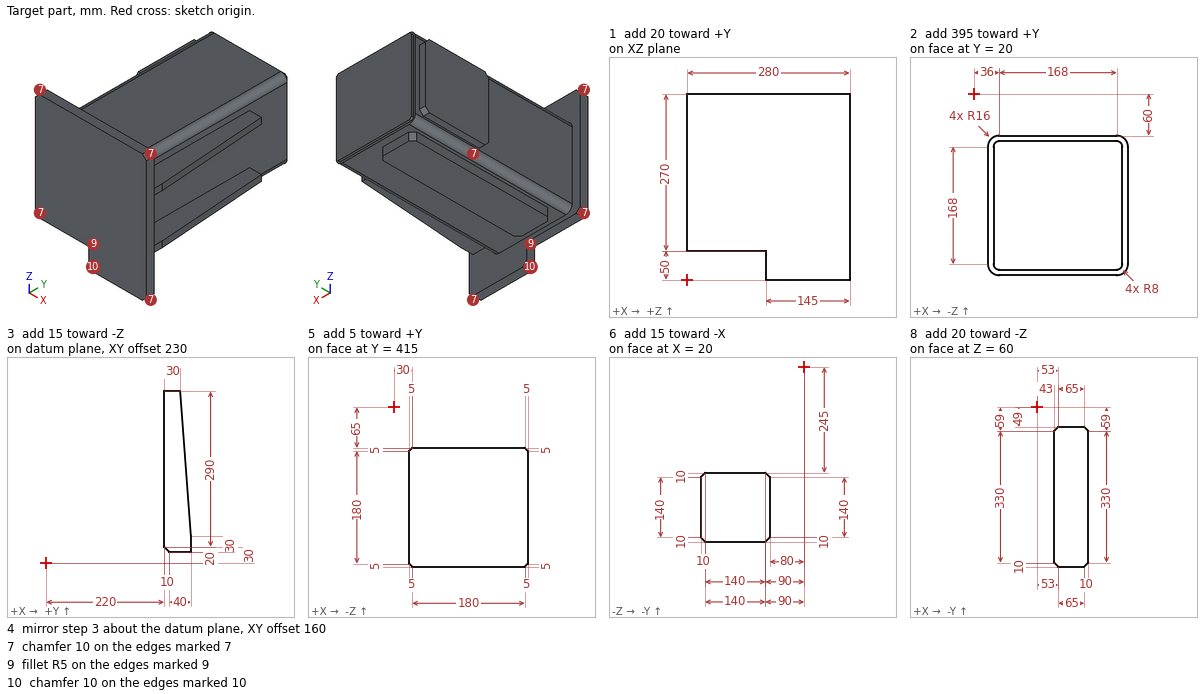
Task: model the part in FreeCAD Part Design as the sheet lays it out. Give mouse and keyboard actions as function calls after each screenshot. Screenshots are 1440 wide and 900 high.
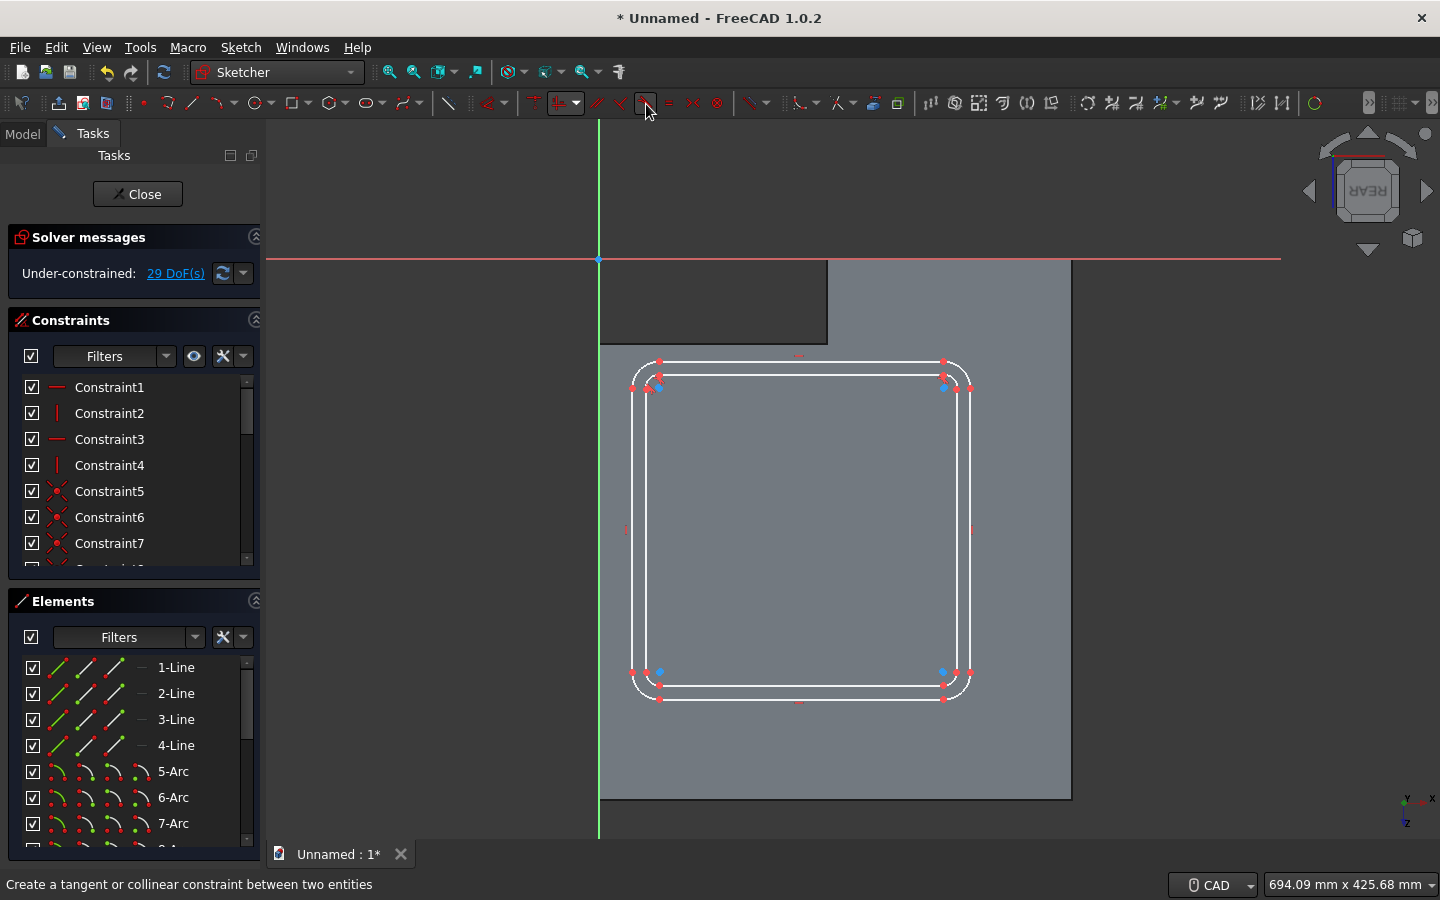
click(632, 474)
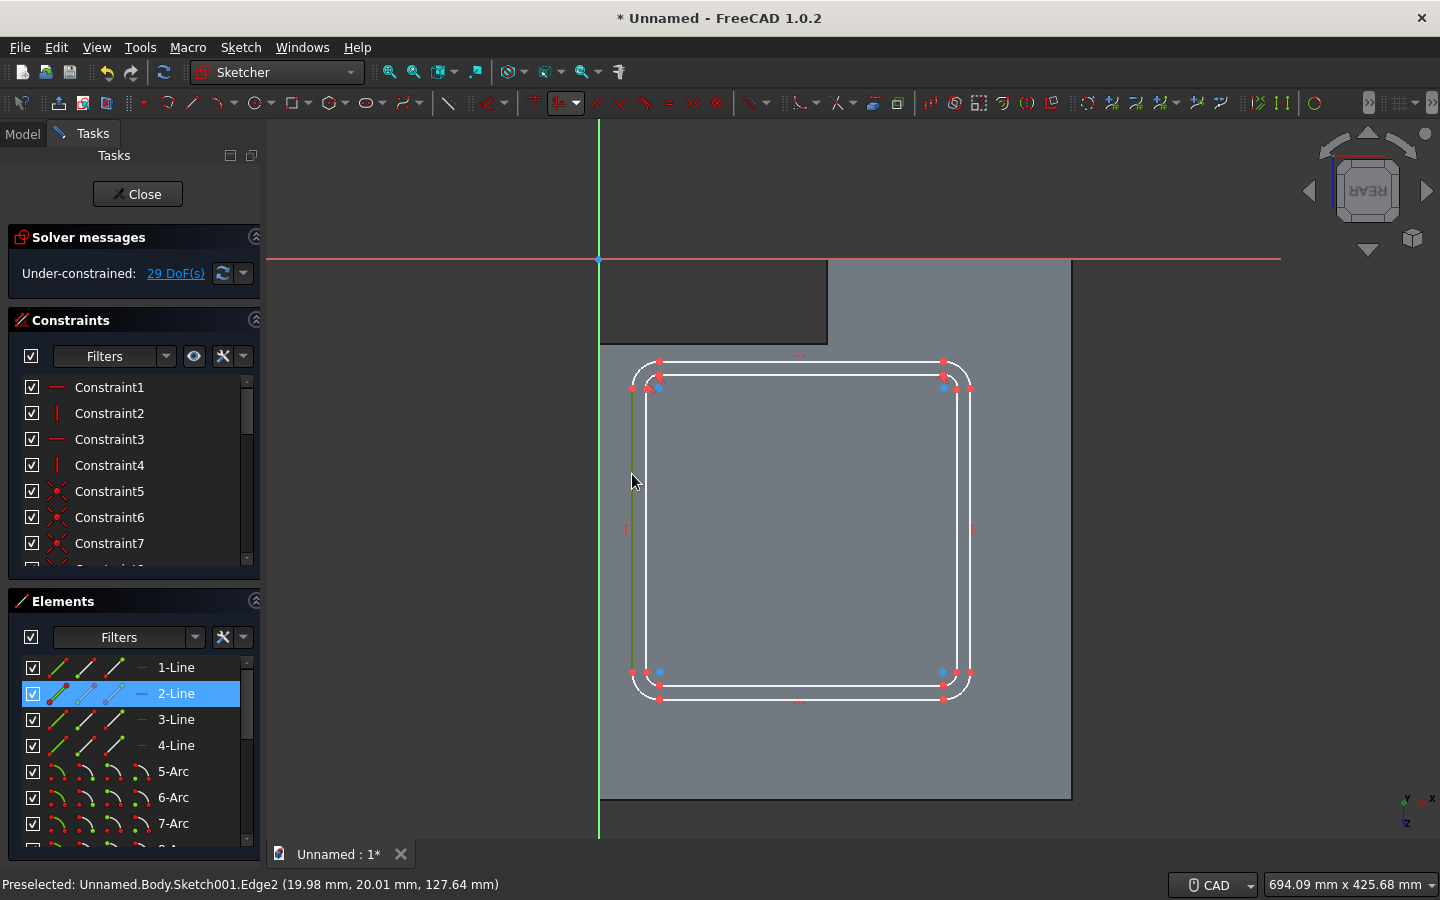
click(635, 685)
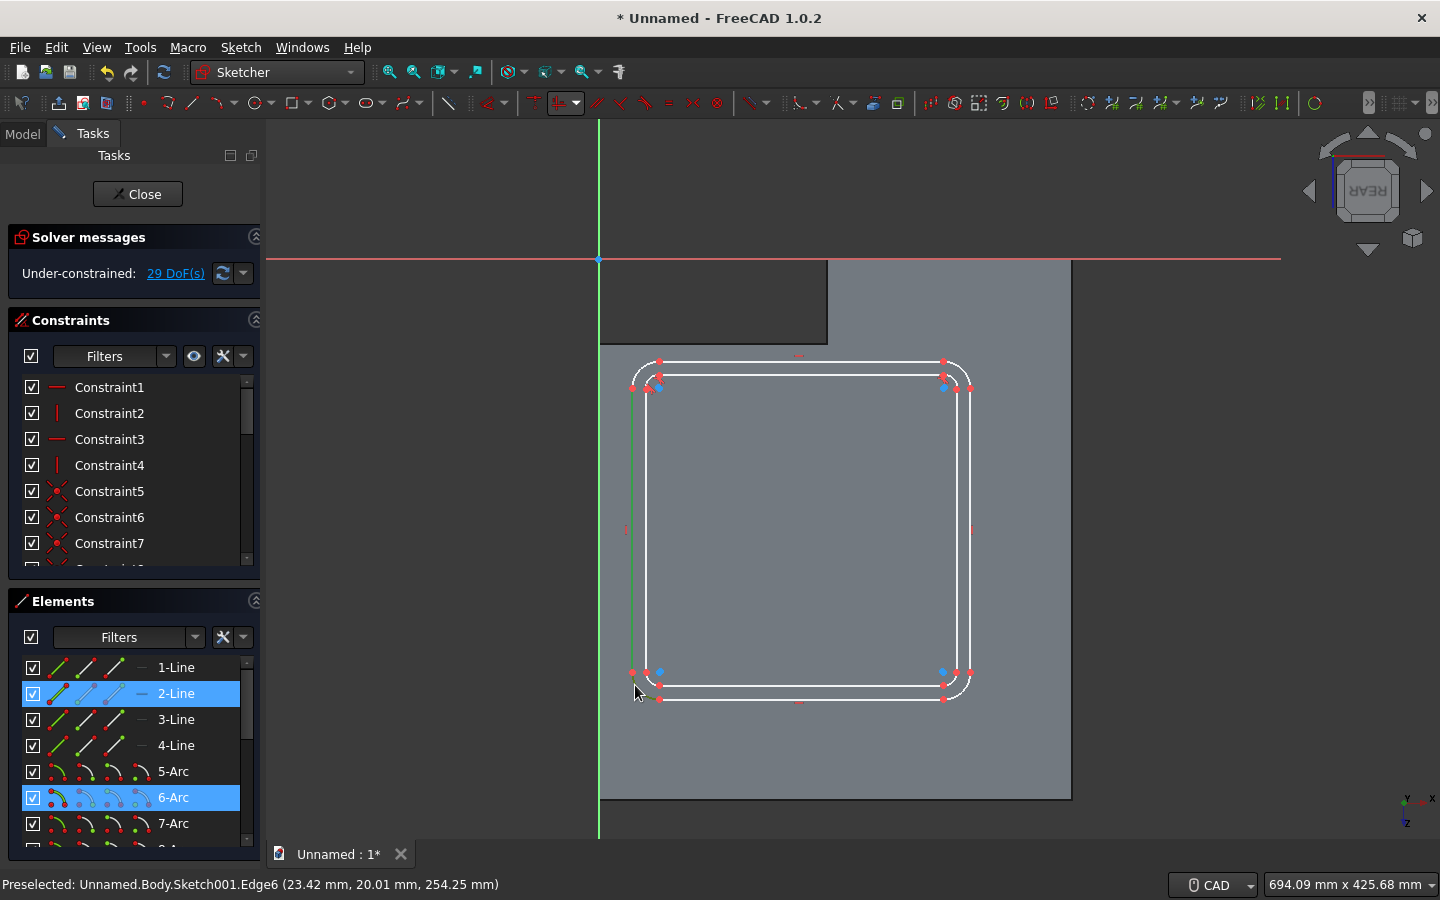
click(646, 104)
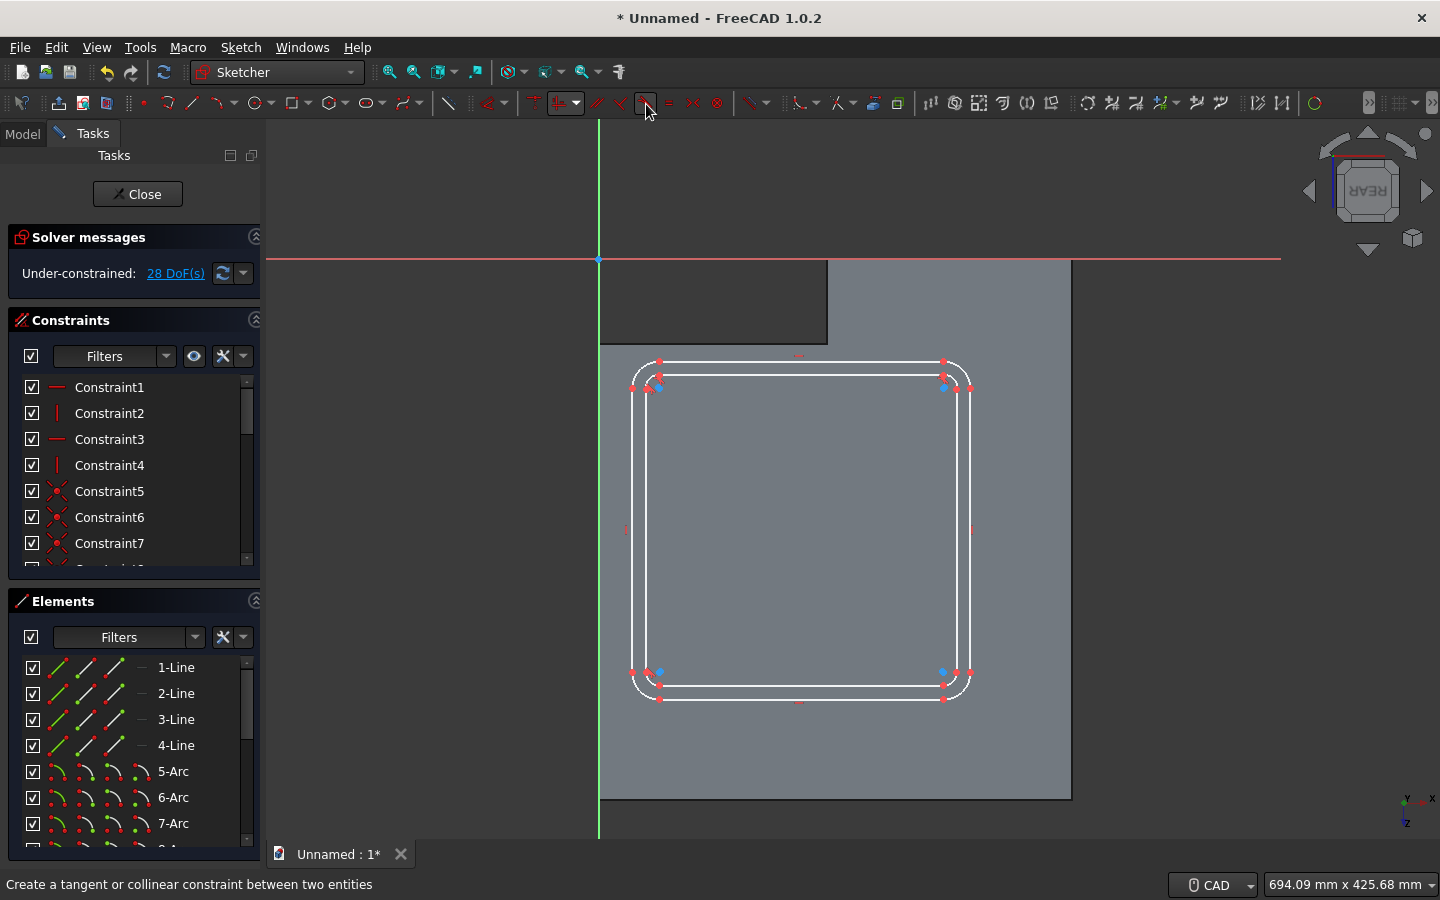
click(745, 700)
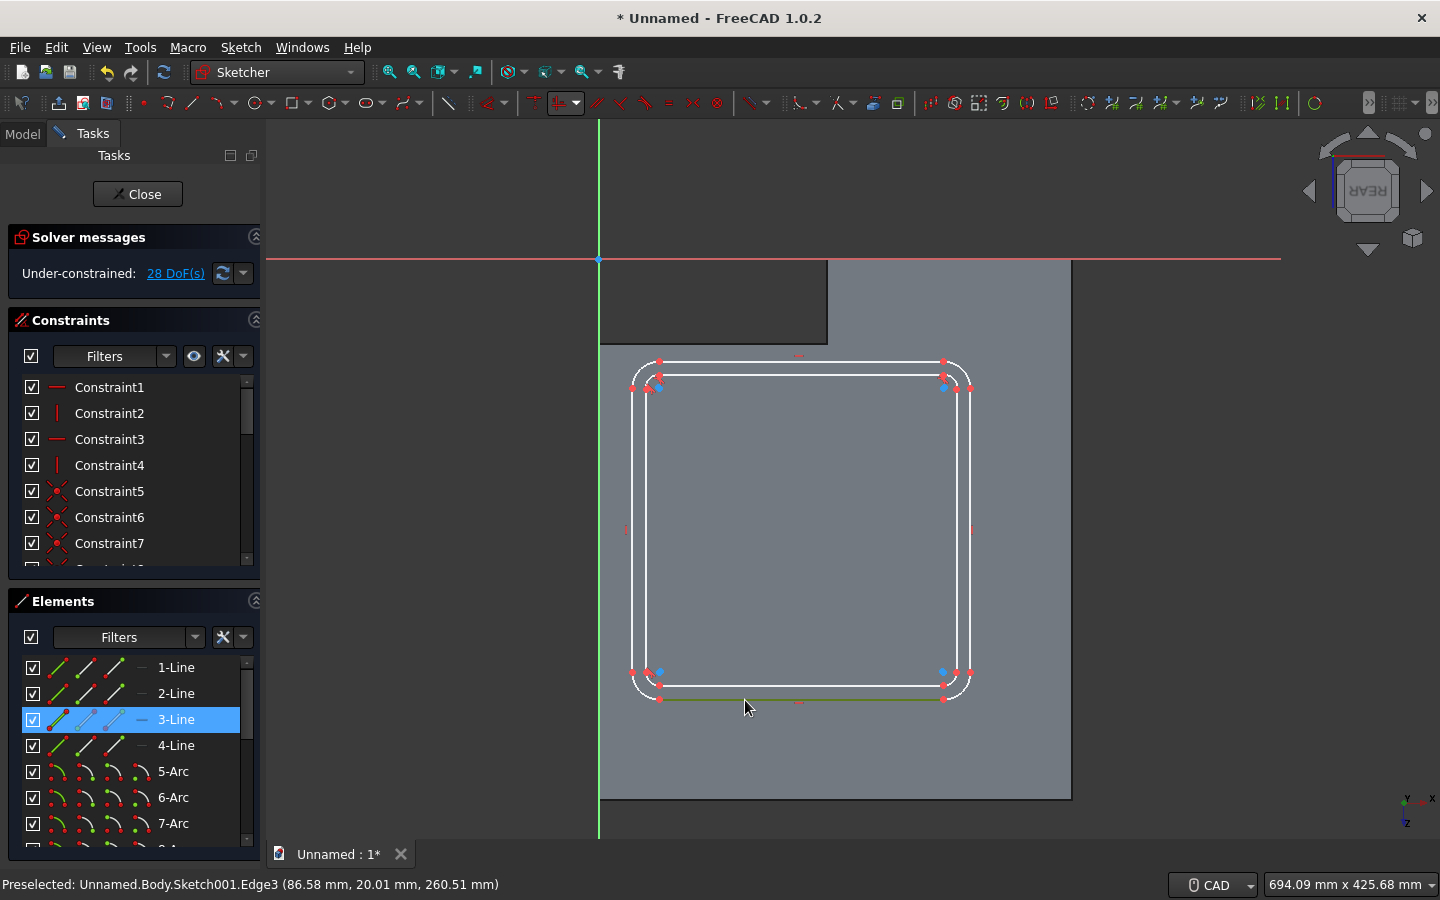
click(635, 685)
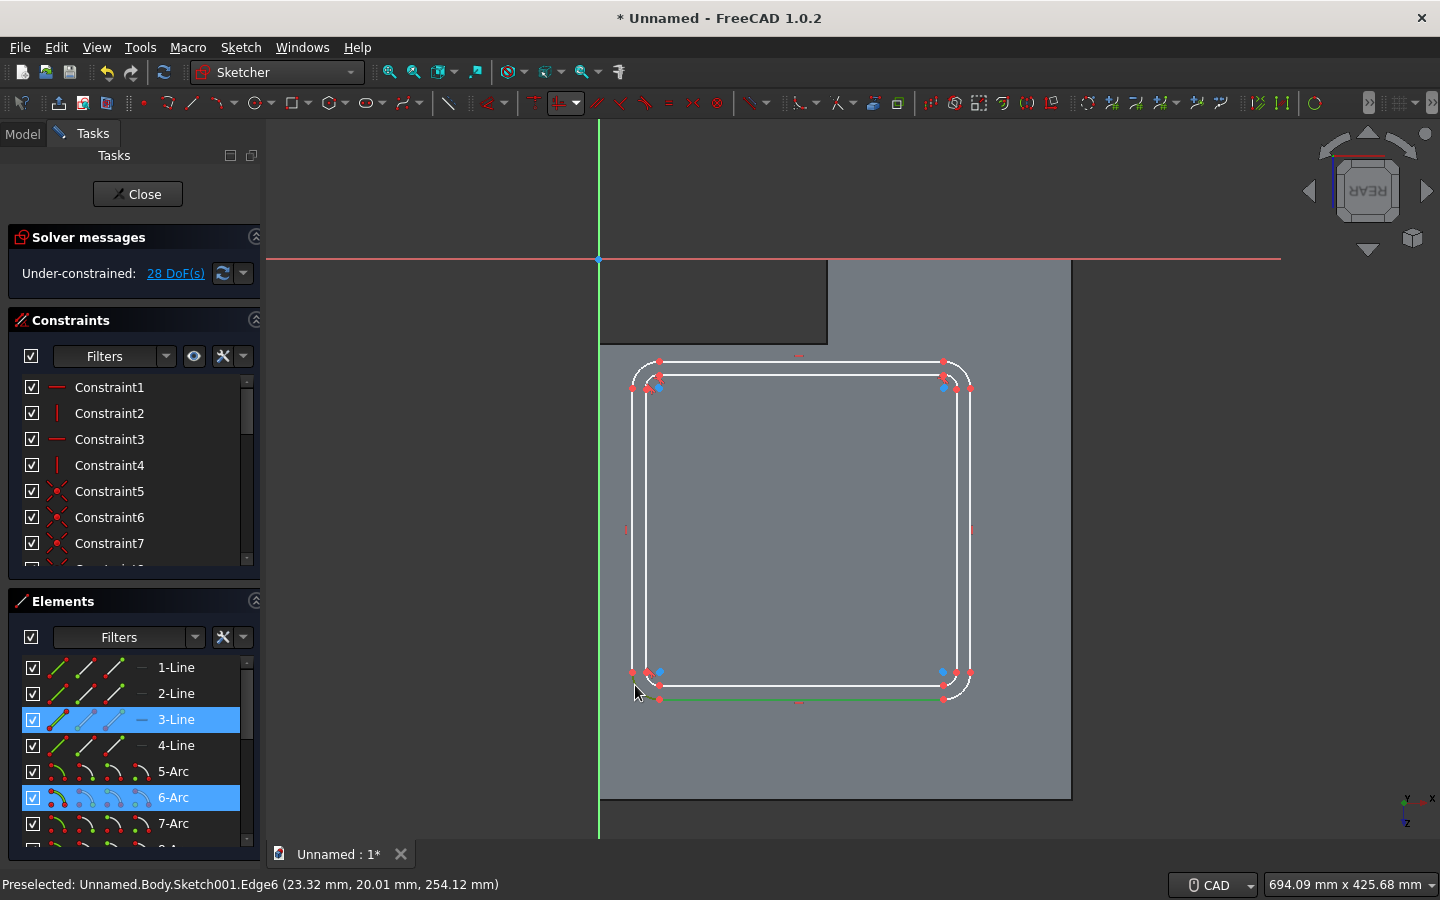
click(646, 104)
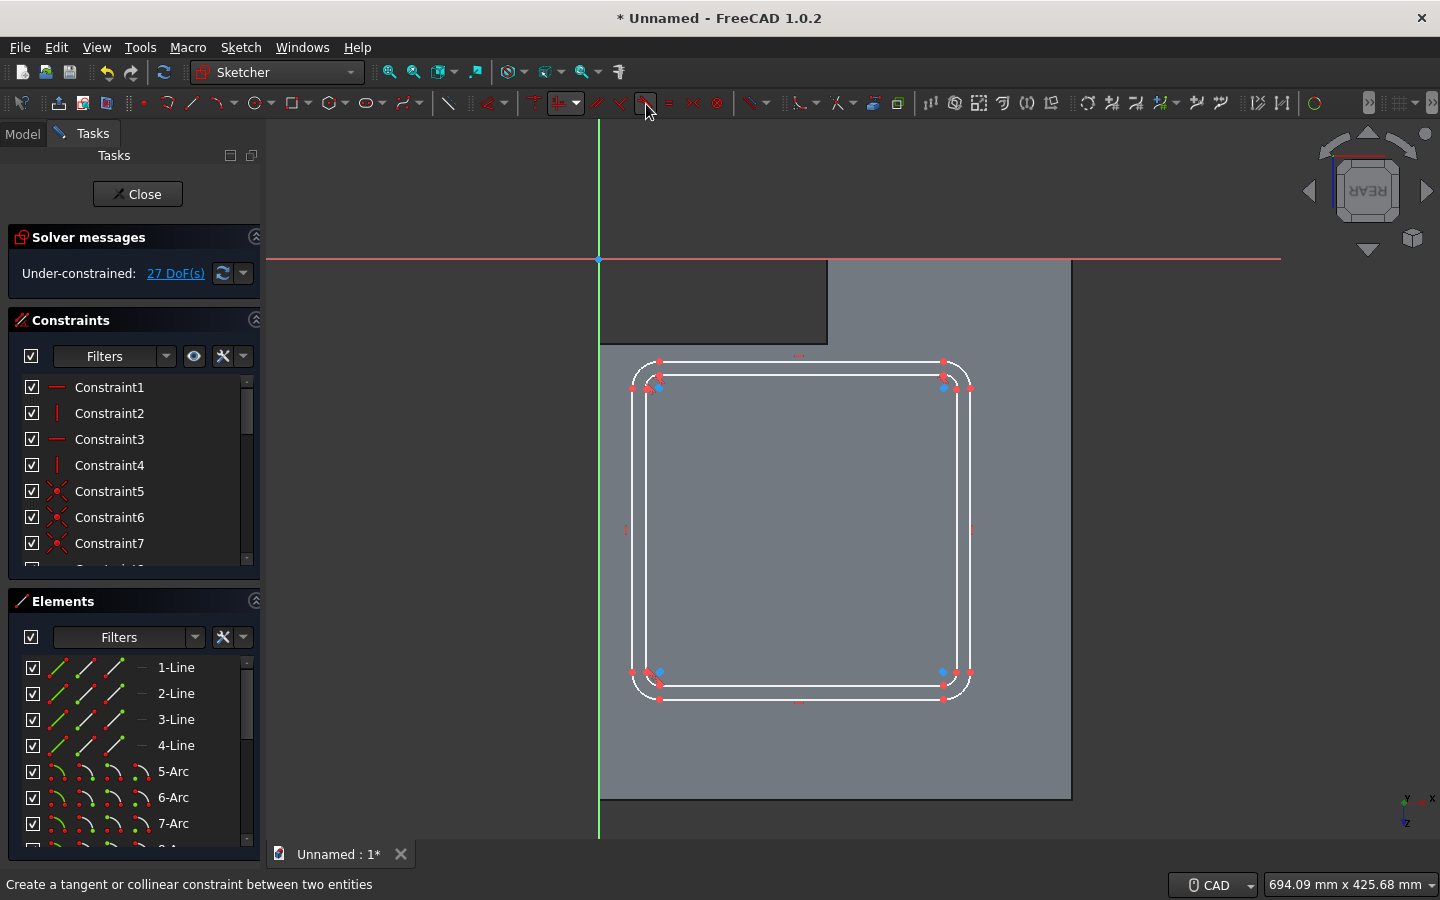
click(745, 700)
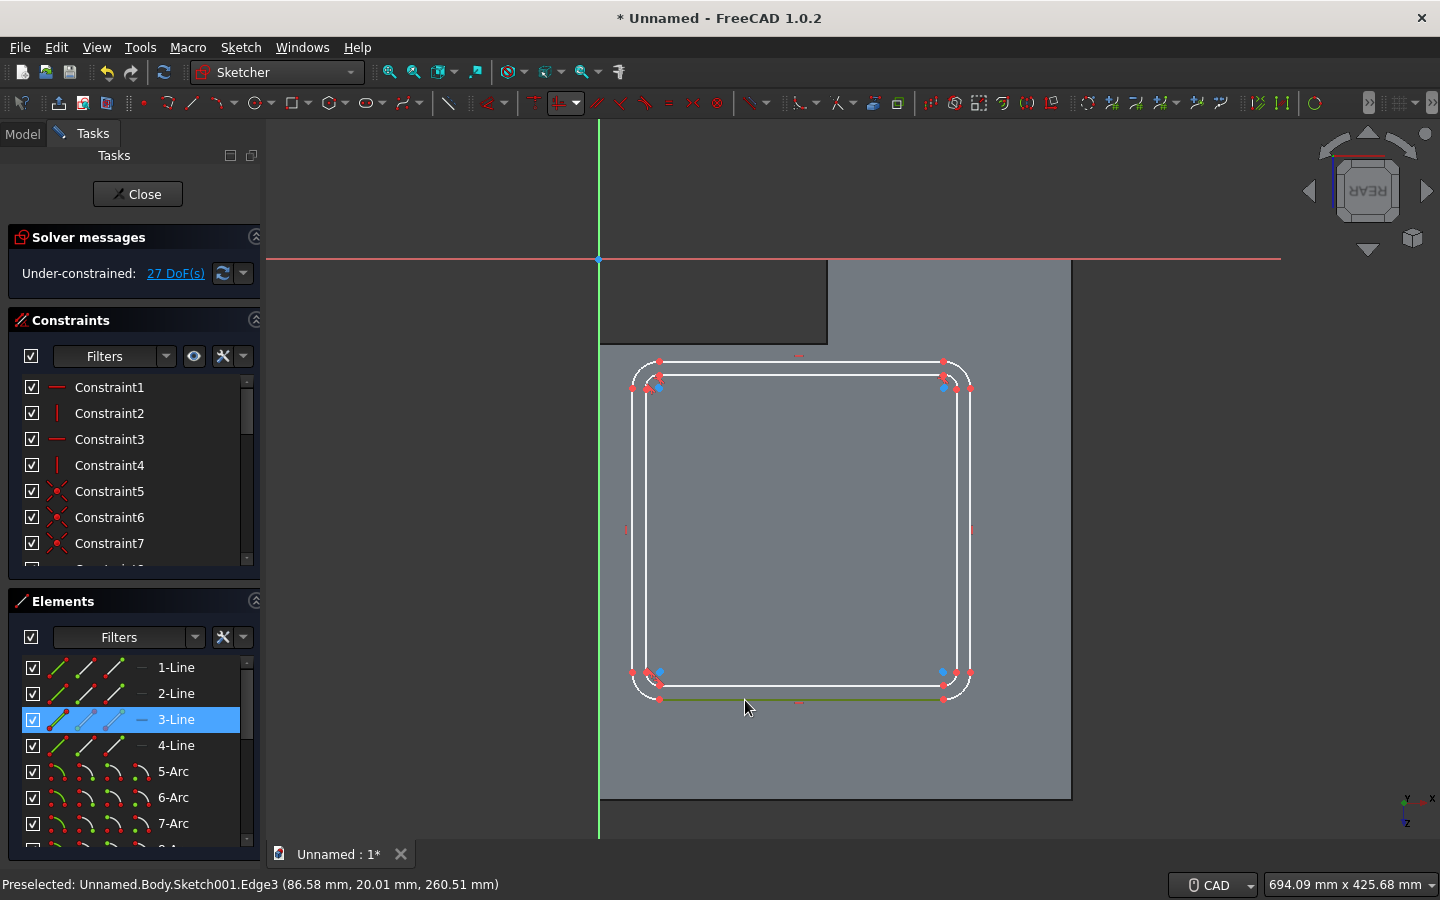
click(956, 697)